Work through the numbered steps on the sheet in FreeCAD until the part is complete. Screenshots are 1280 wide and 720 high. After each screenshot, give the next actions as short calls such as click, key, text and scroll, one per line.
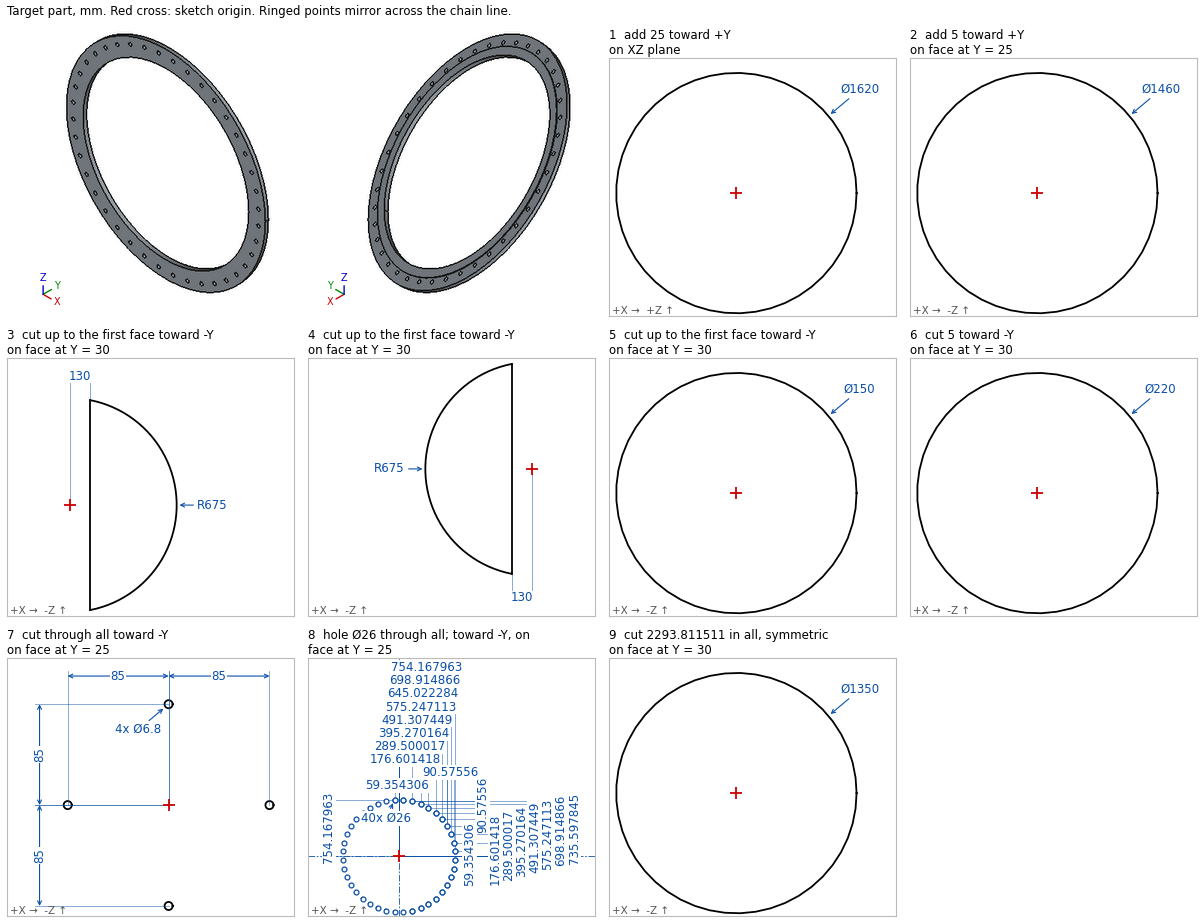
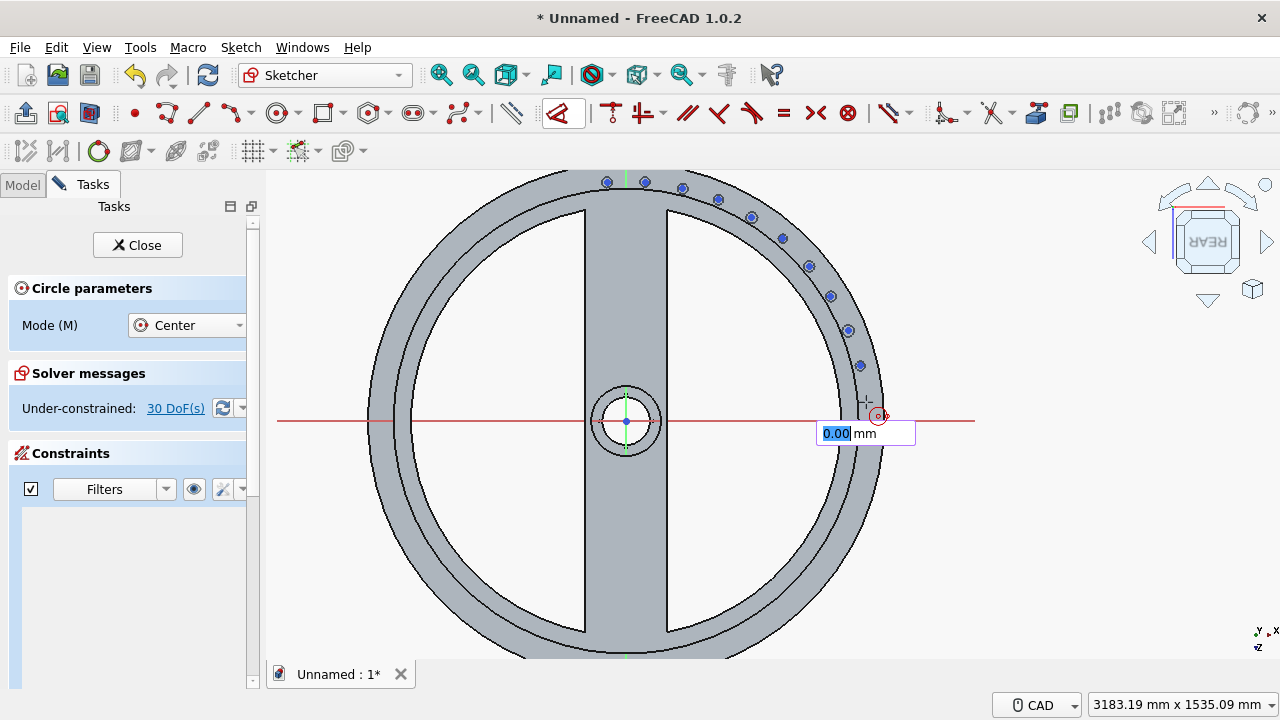
scroll(869, 399, up, 7)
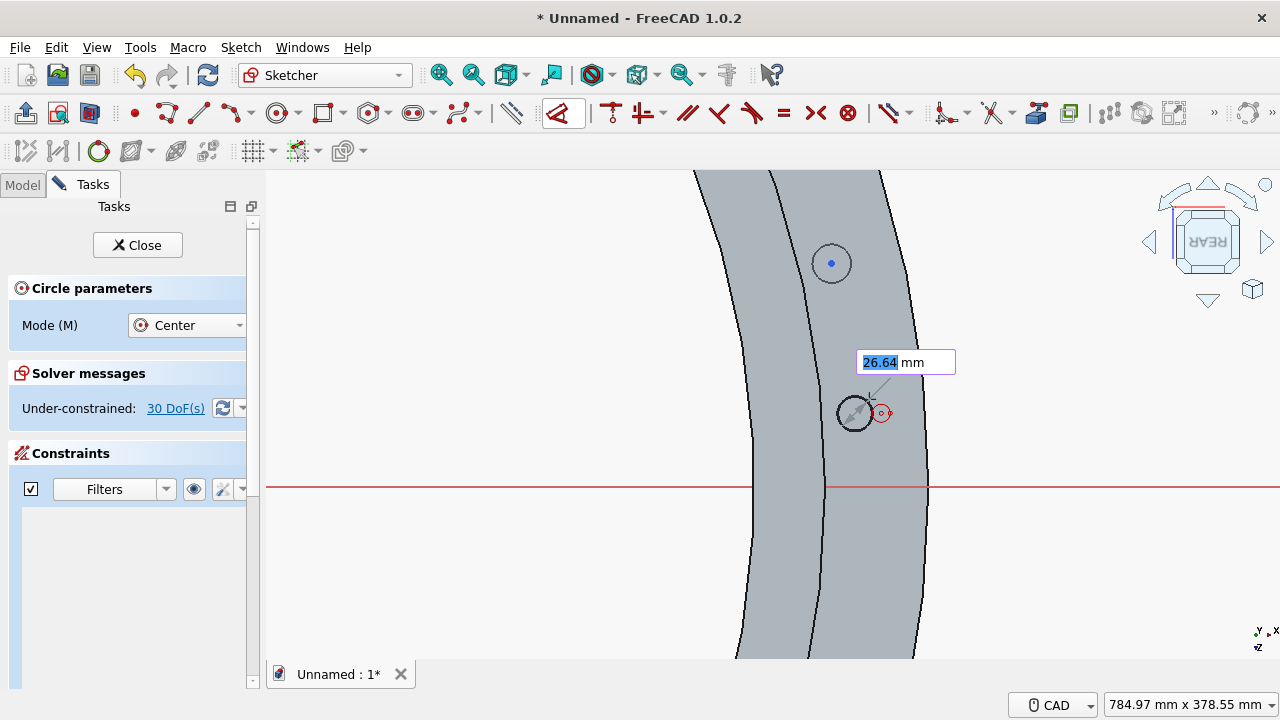
click(868, 399)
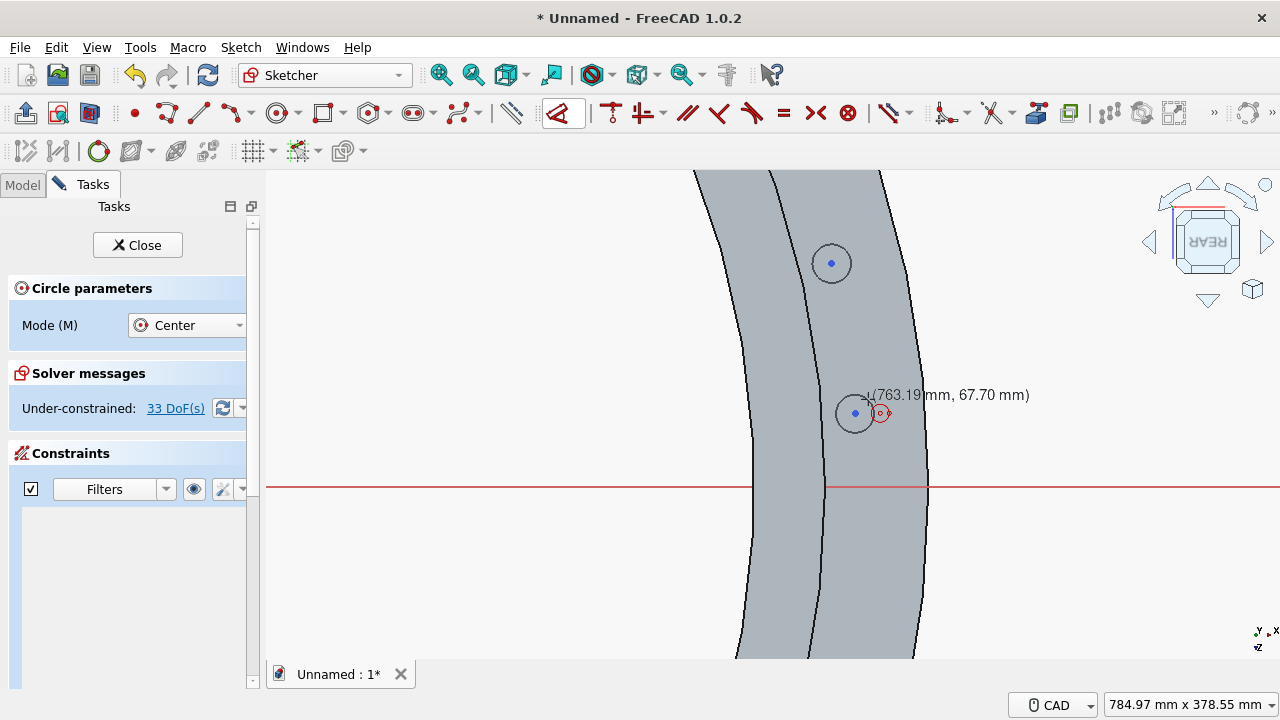
scroll(856, 564, up, 2)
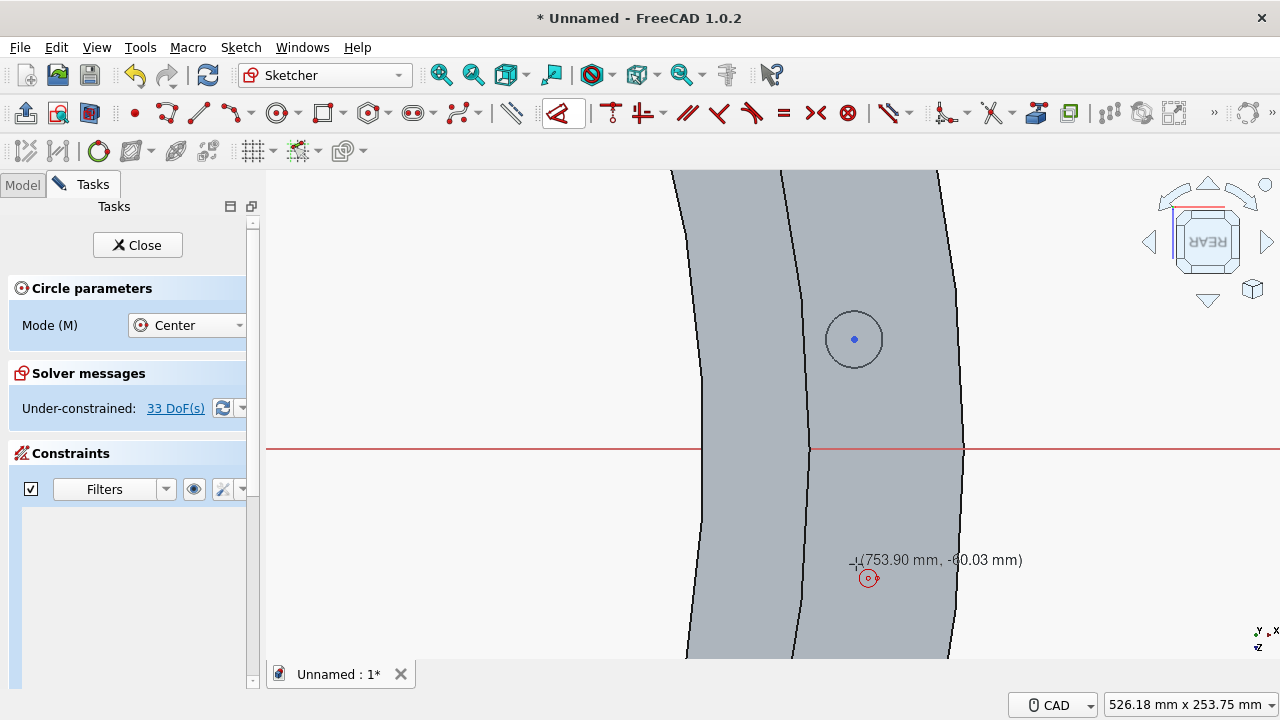
scroll(867, 410, down, 11)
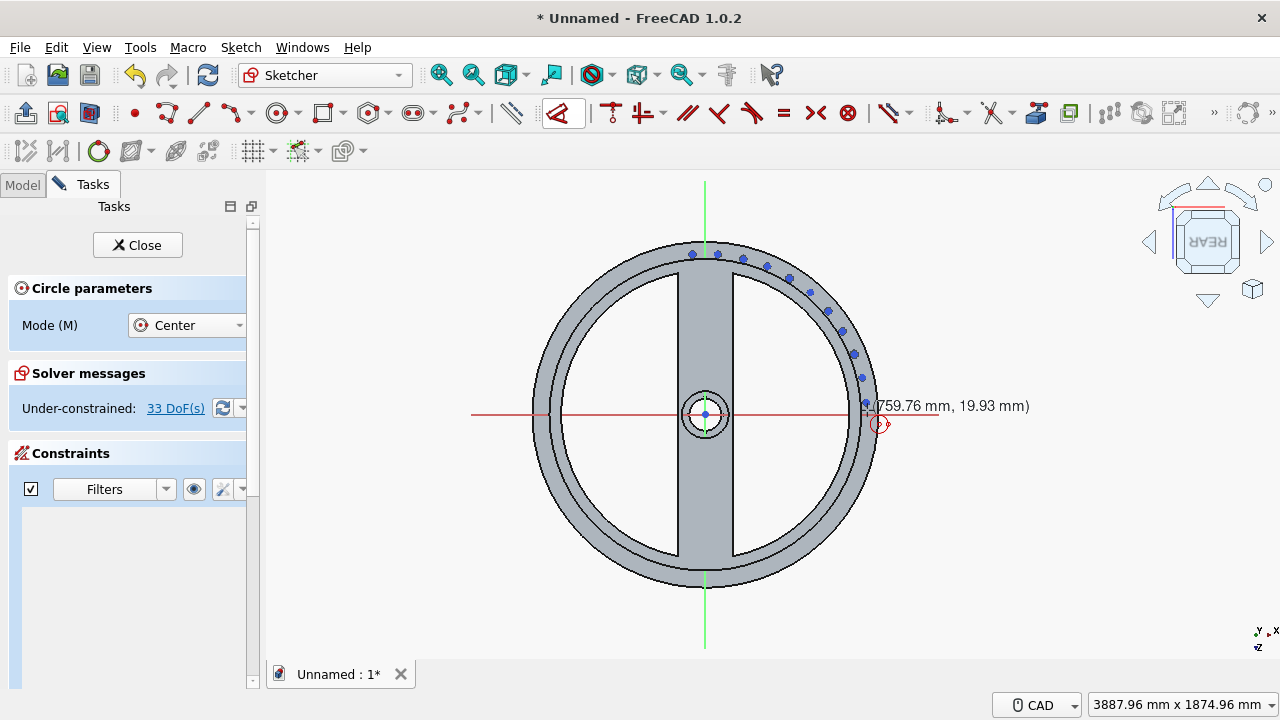
scroll(866, 427, up, 2)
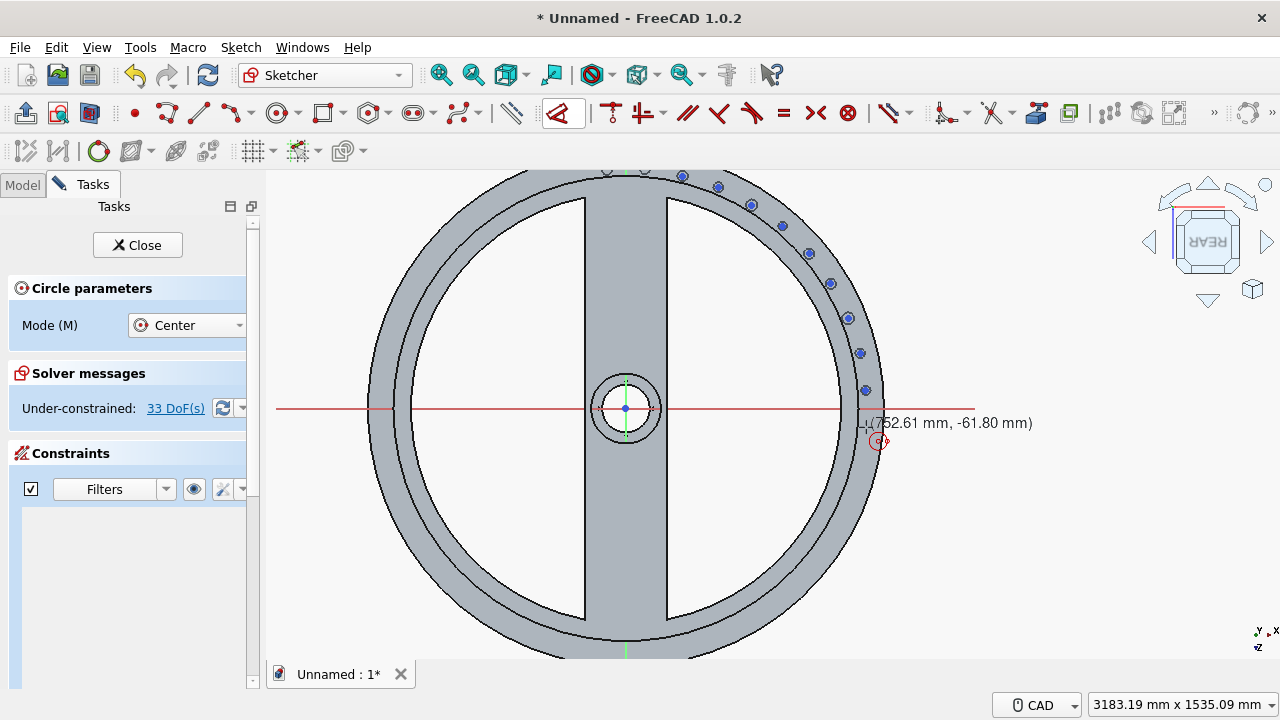
click(866, 427)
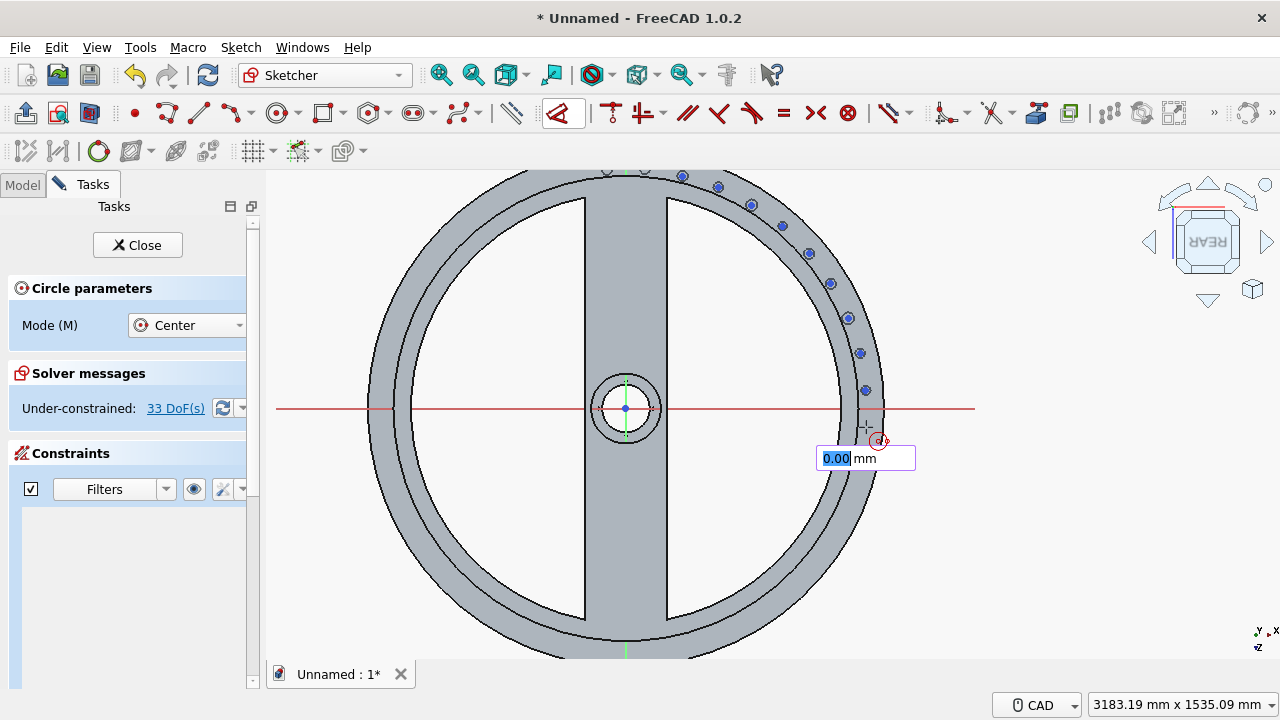
scroll(869, 425, up, 7)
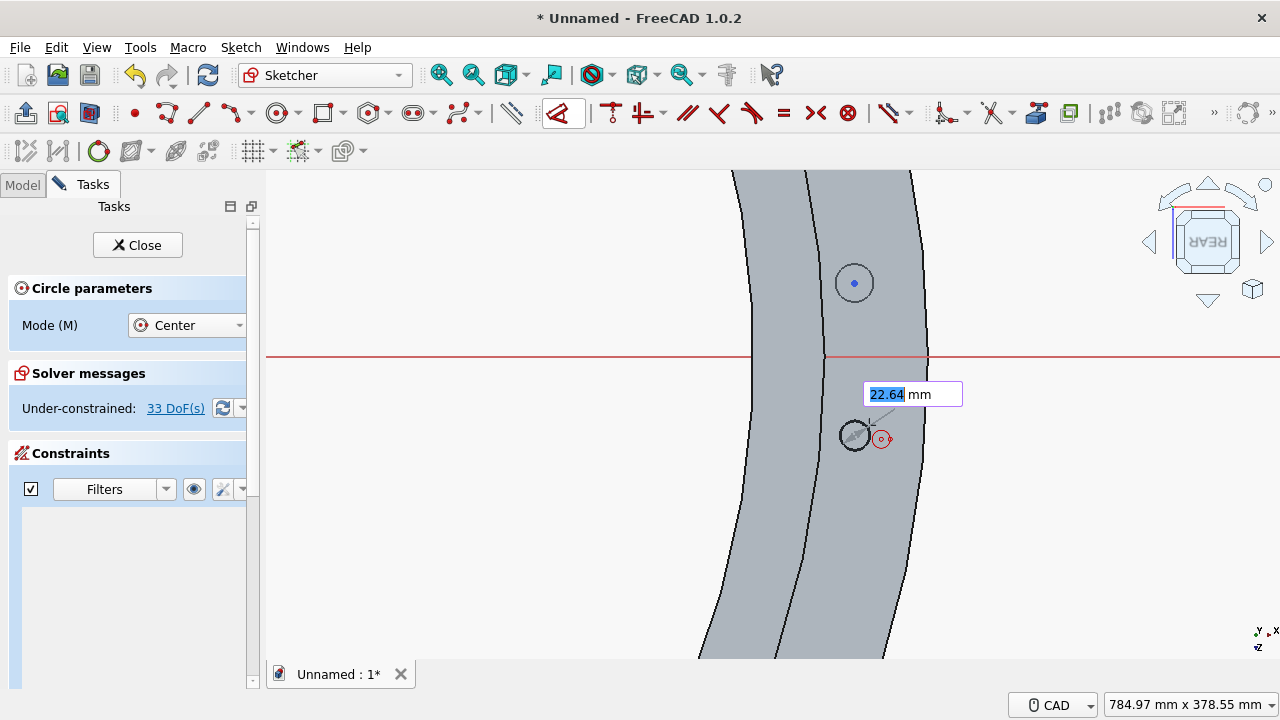
click(868, 421)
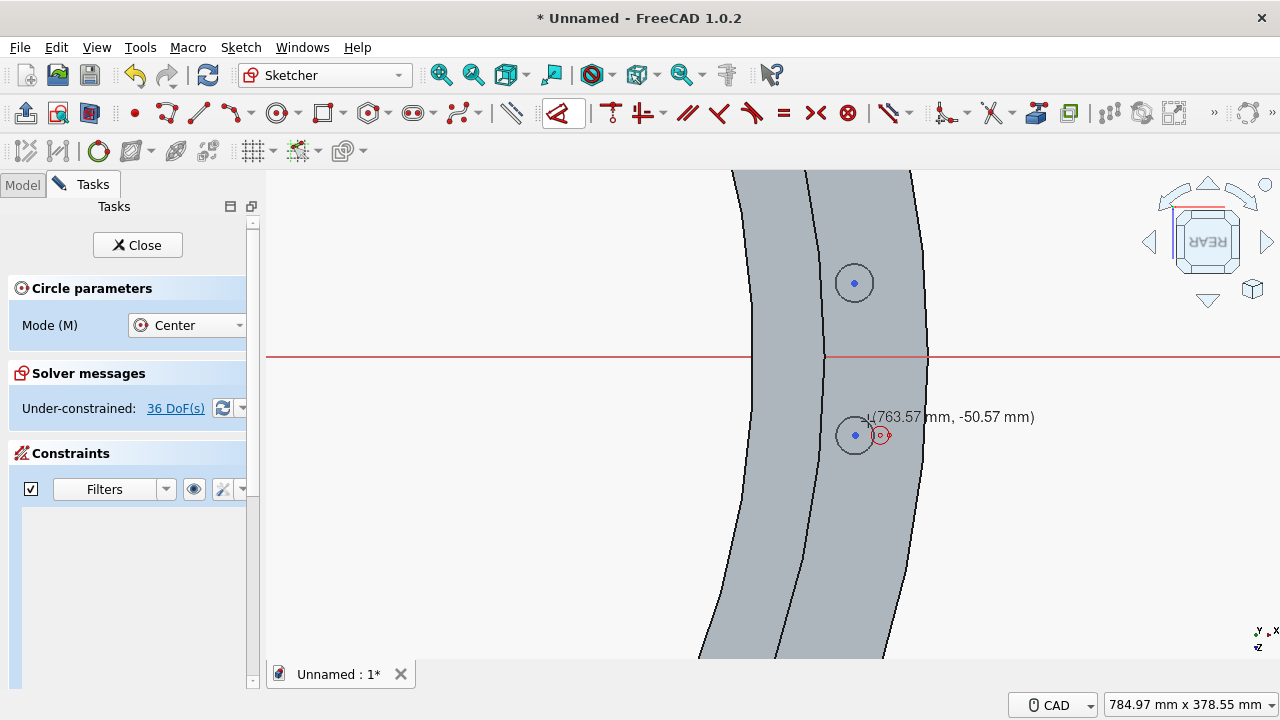
scroll(832, 585, up, 2)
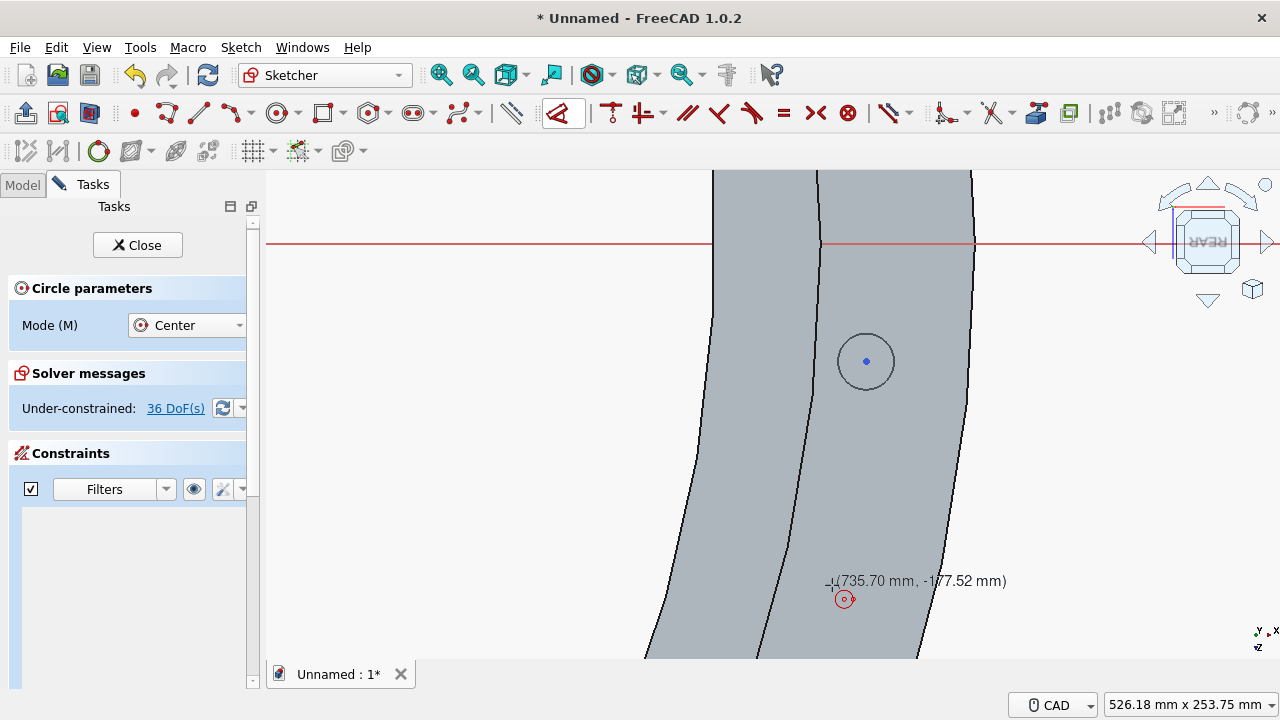
scroll(865, 436, down, 11)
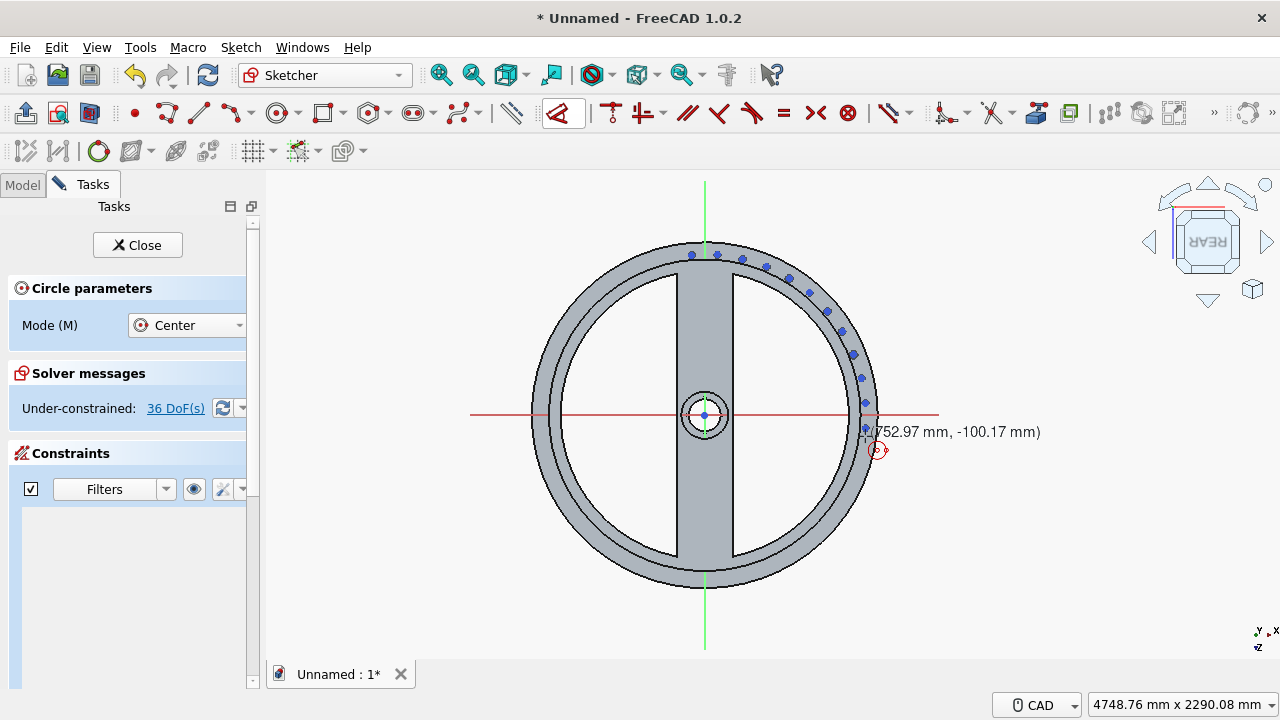
click(862, 453)